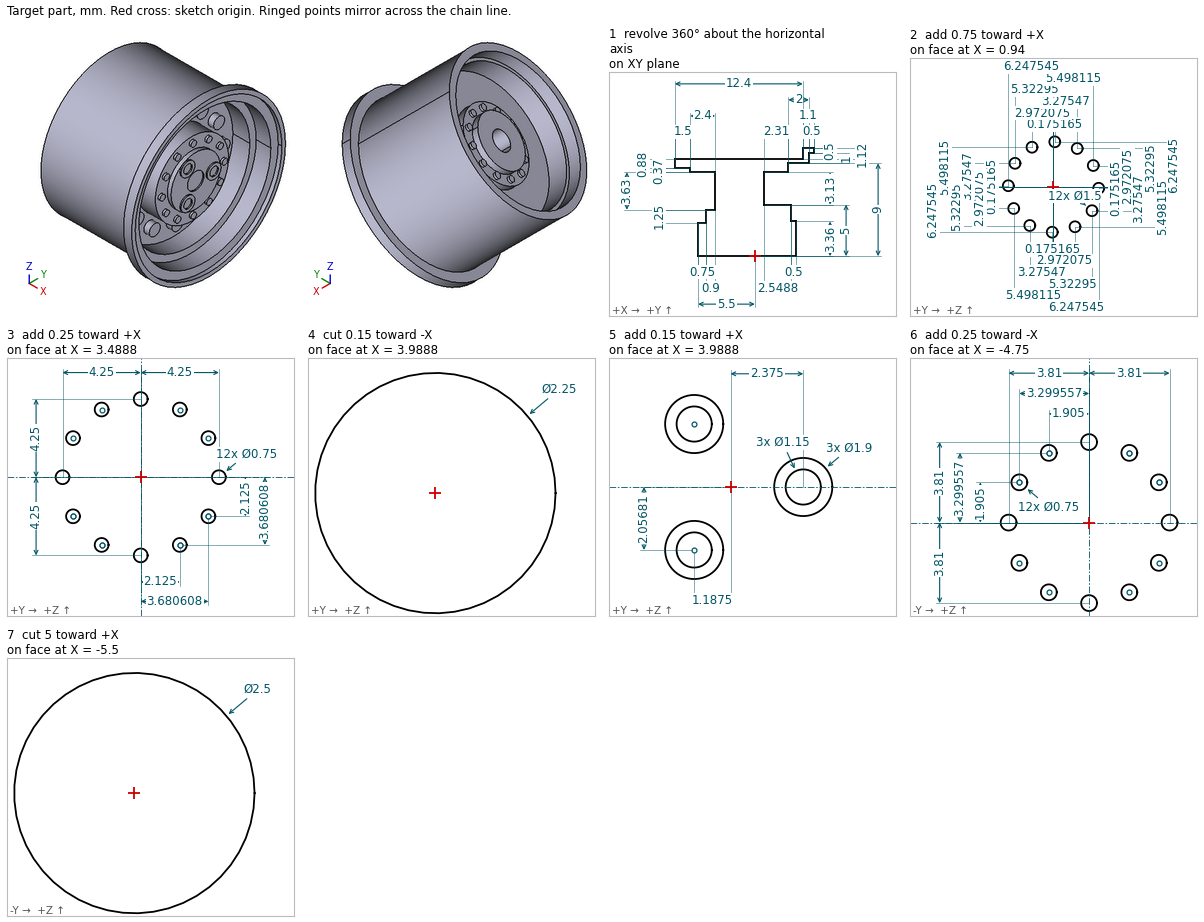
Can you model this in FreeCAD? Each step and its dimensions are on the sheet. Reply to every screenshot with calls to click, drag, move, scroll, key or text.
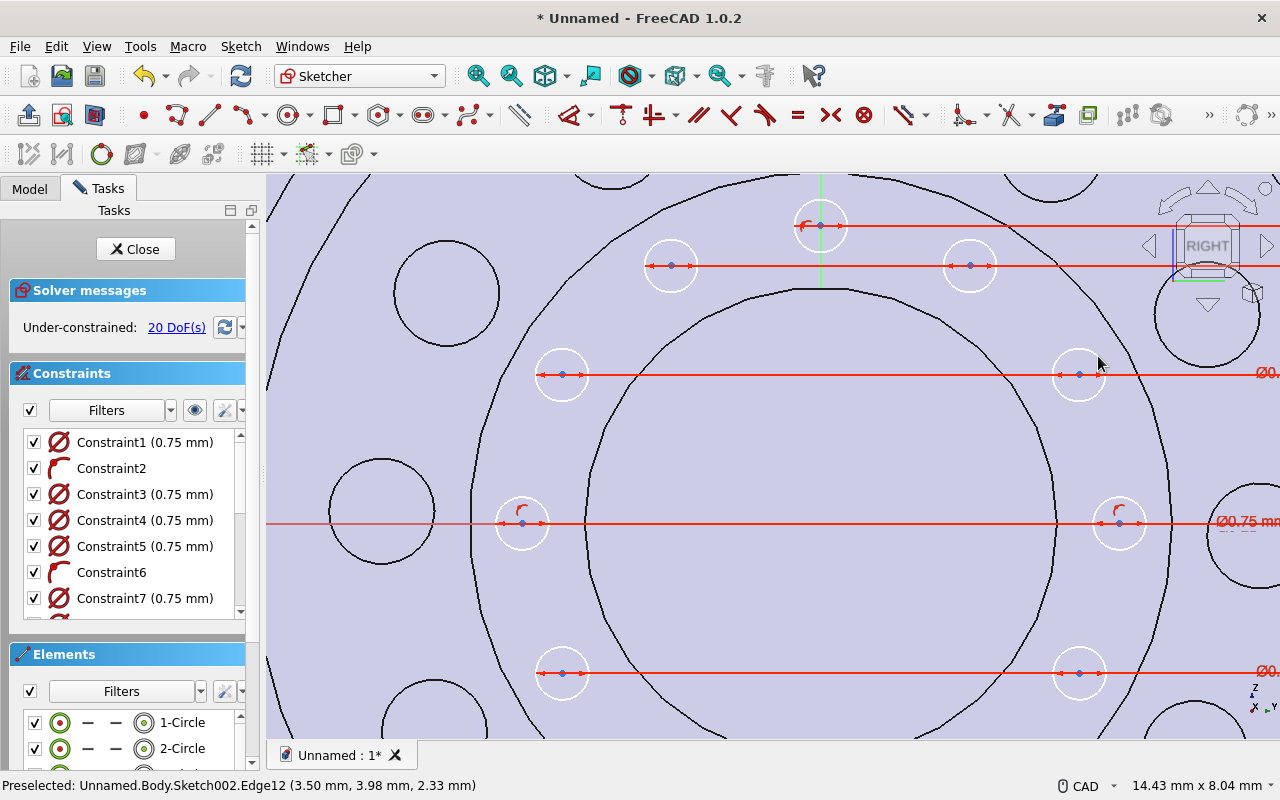
scroll(563, 375, down, 3)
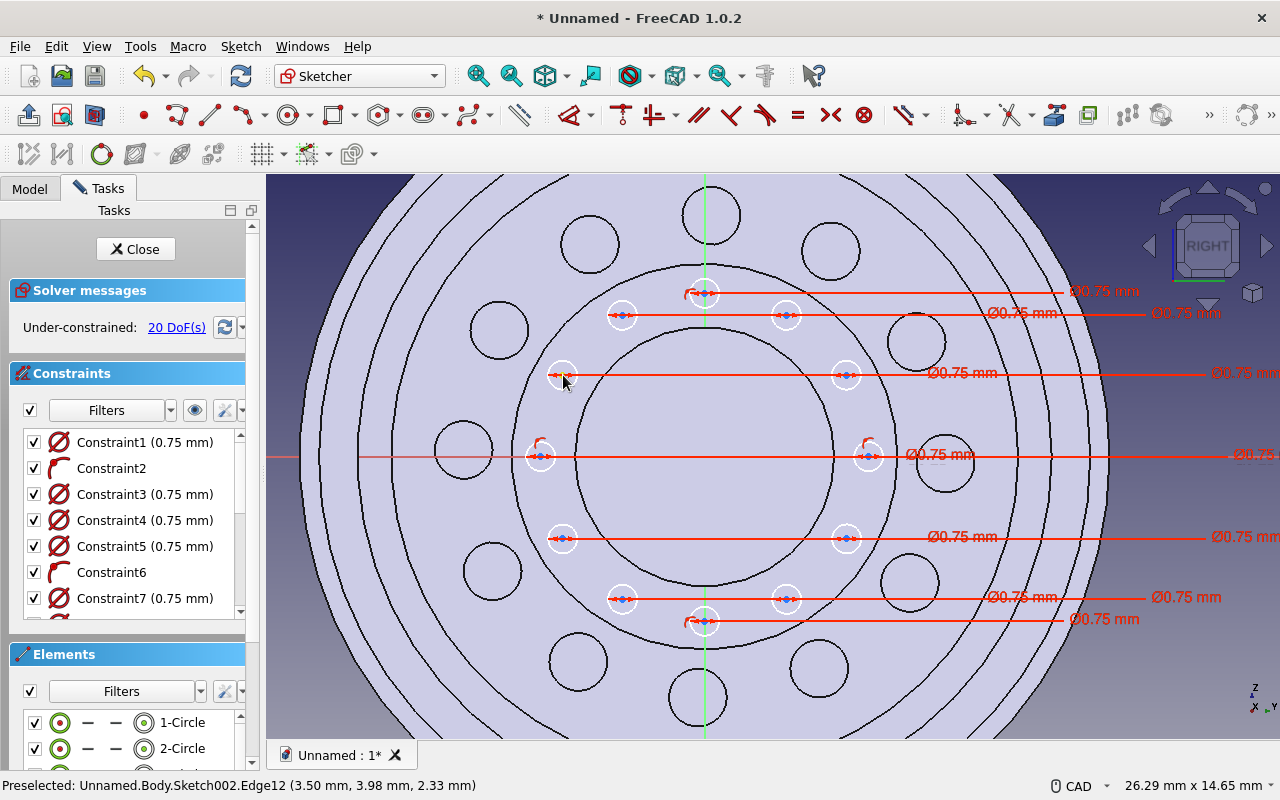
click(787, 599)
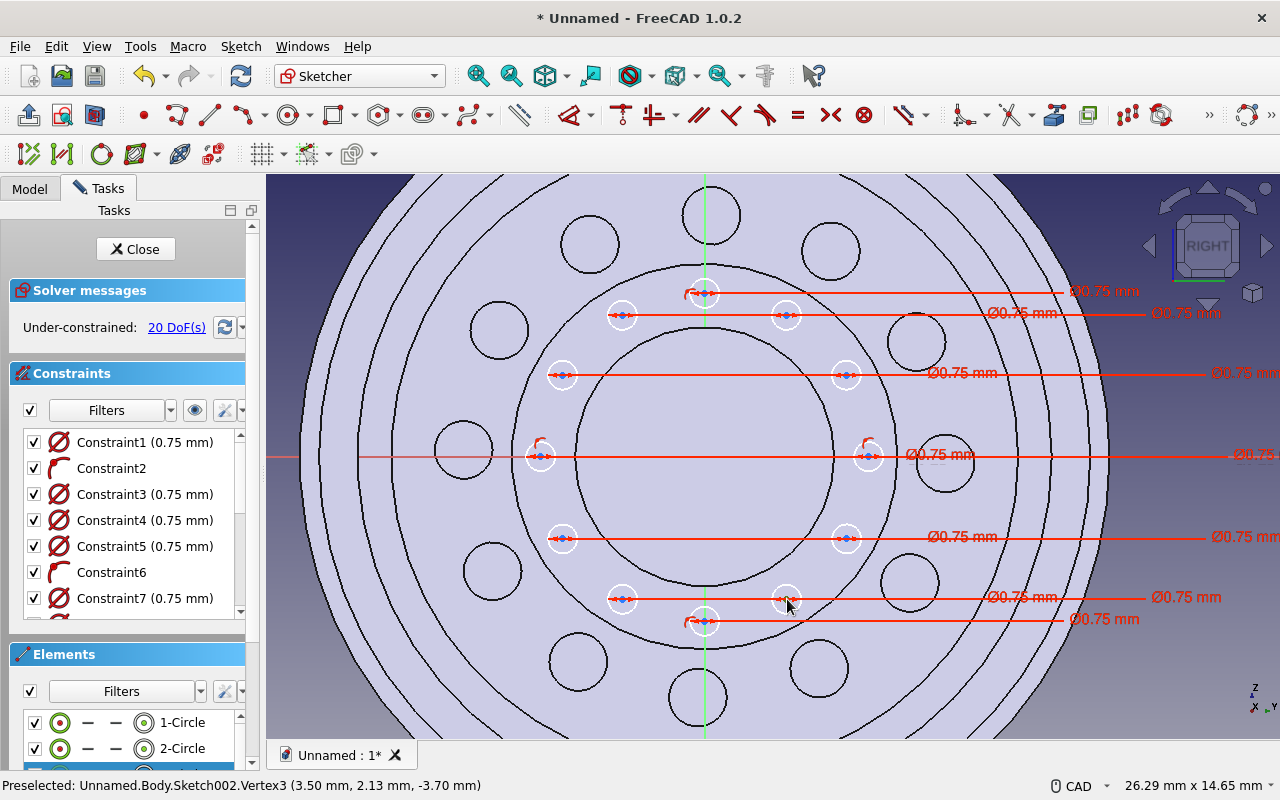
click(623, 599)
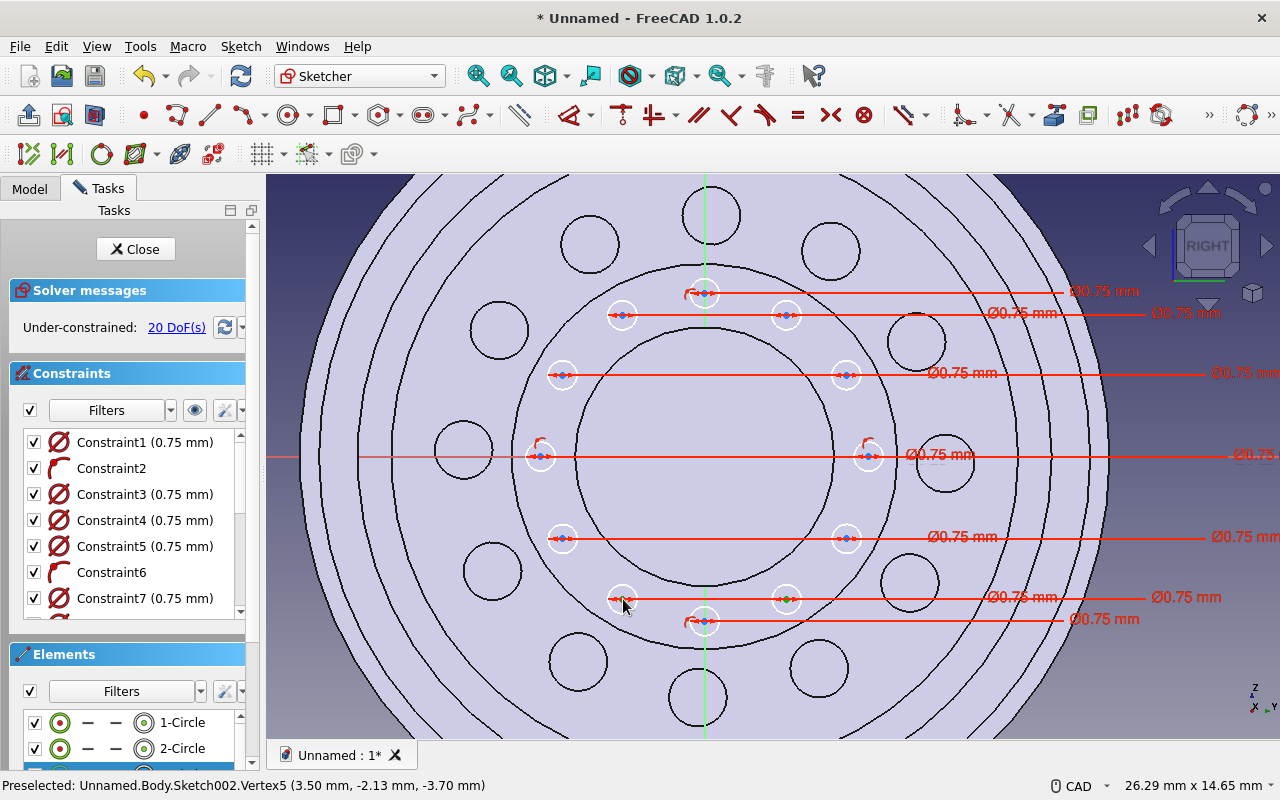
click(705, 675)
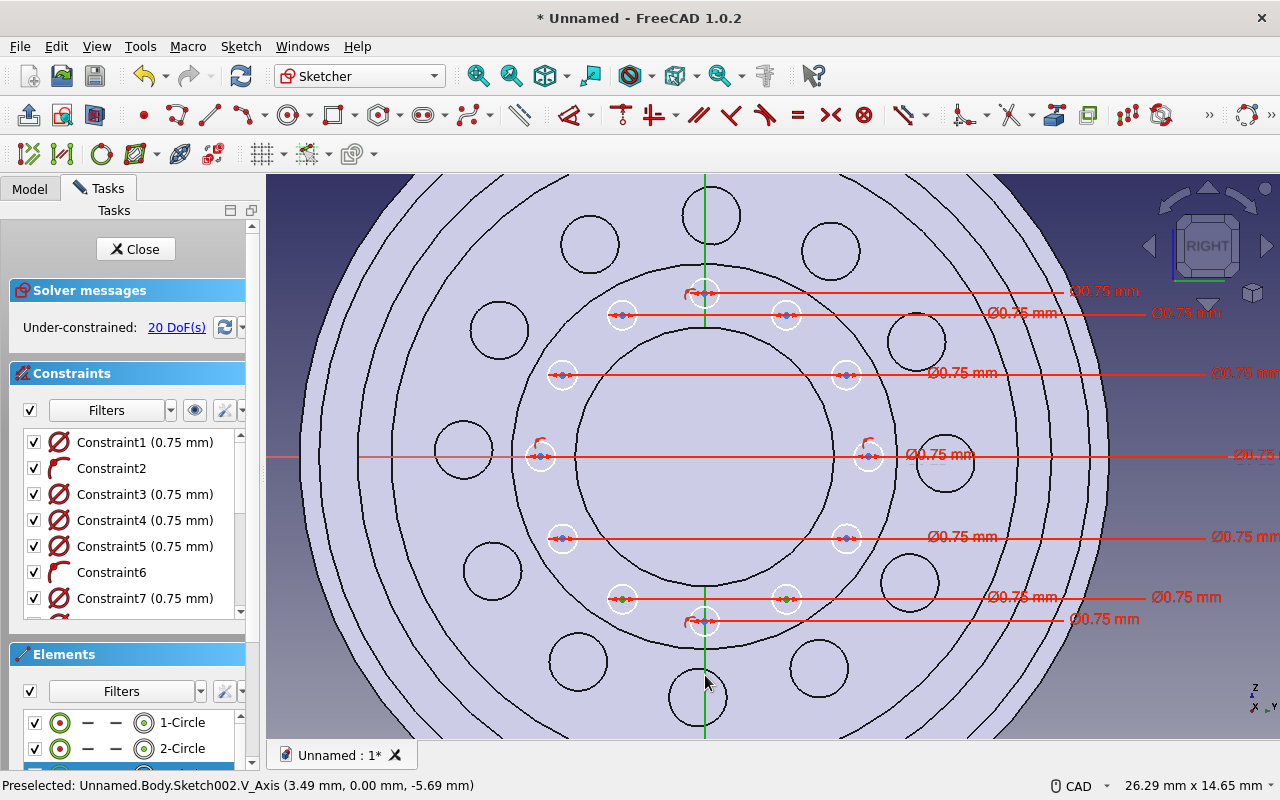
click(831, 116)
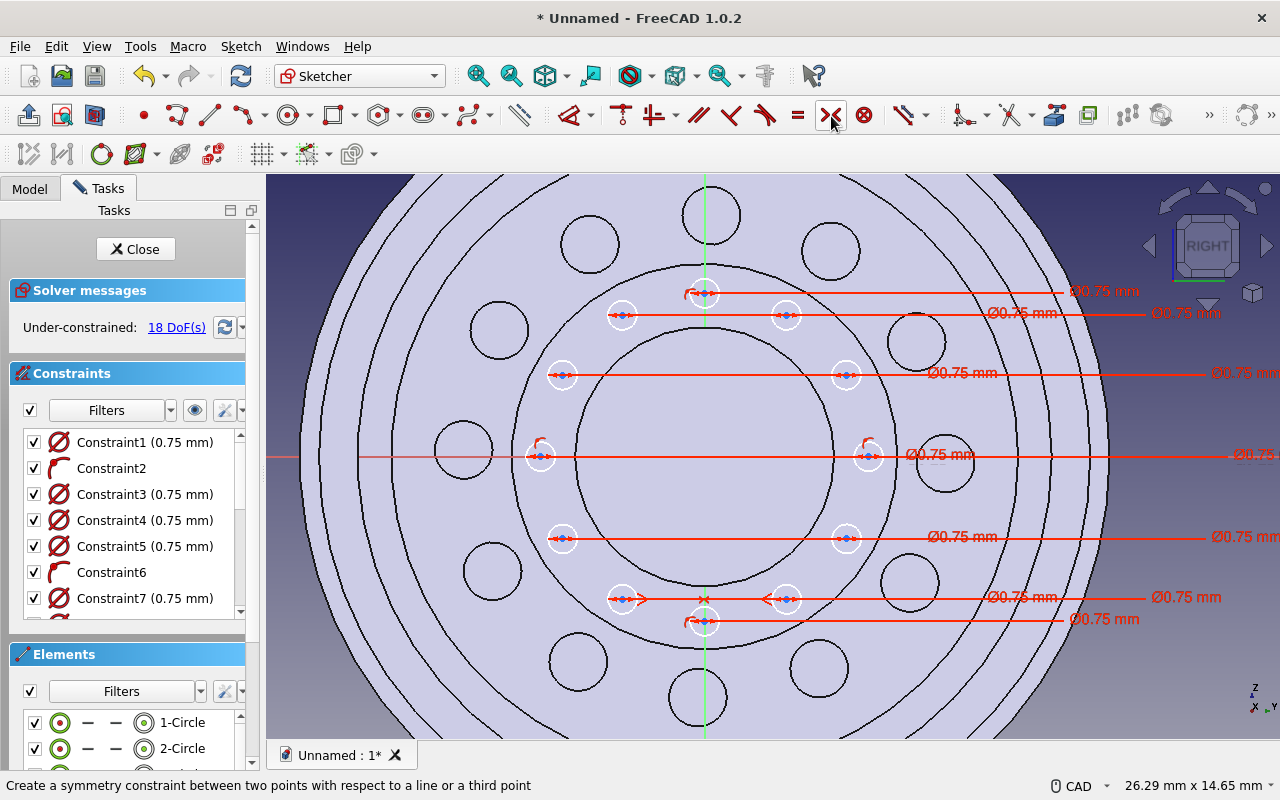
click(847, 539)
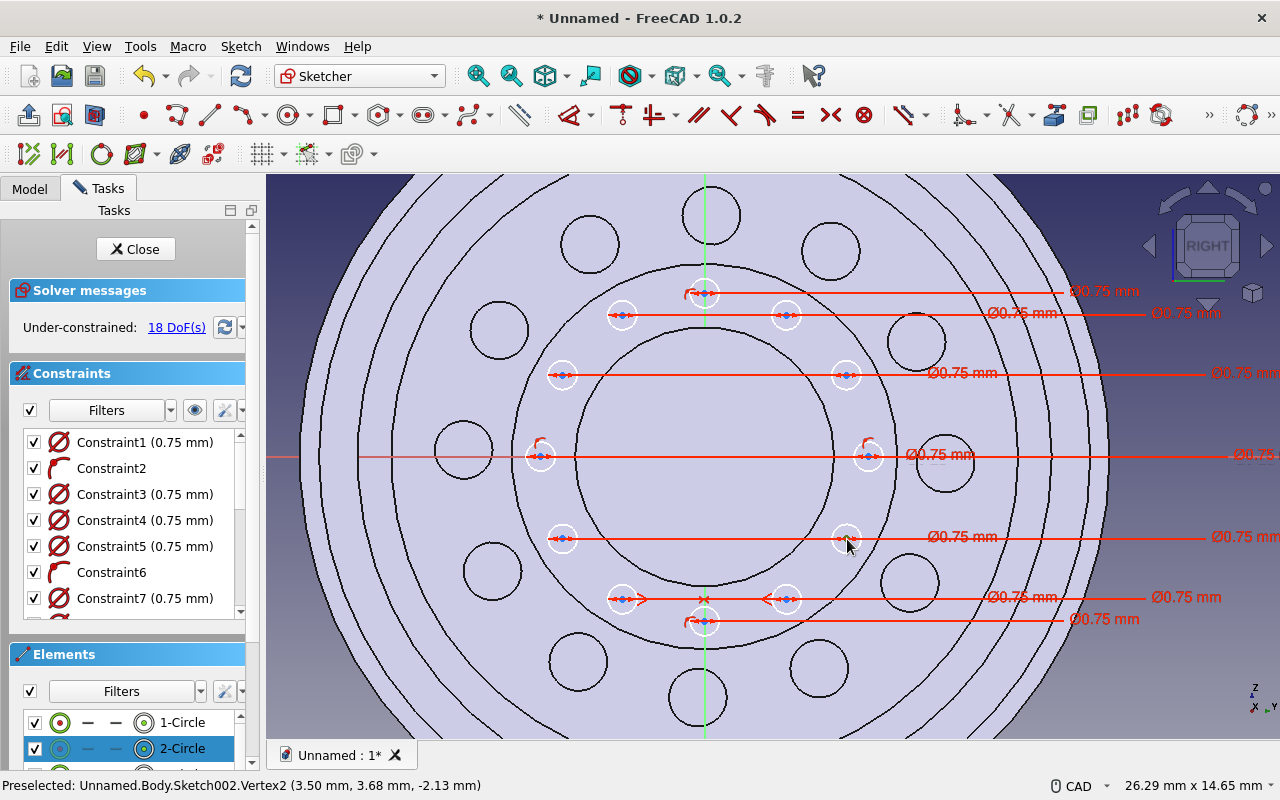
click(563, 539)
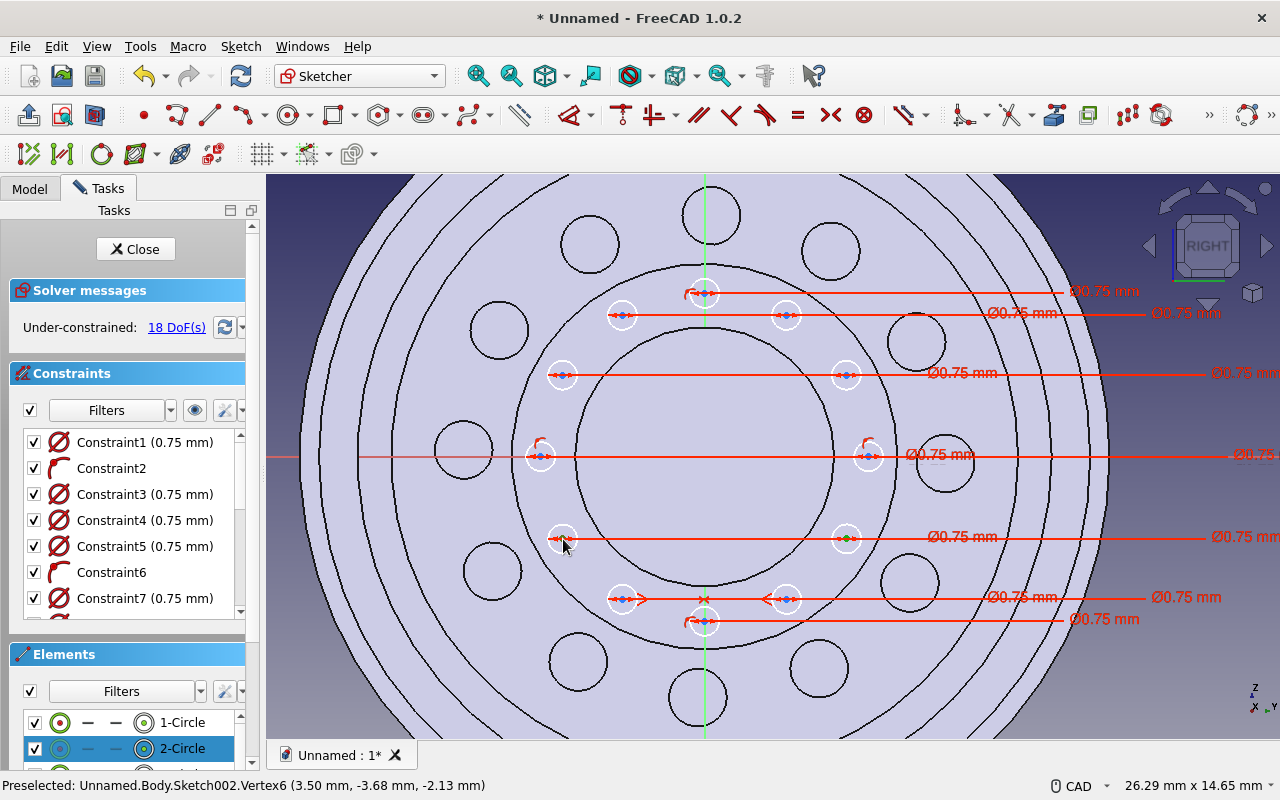
click(705, 675)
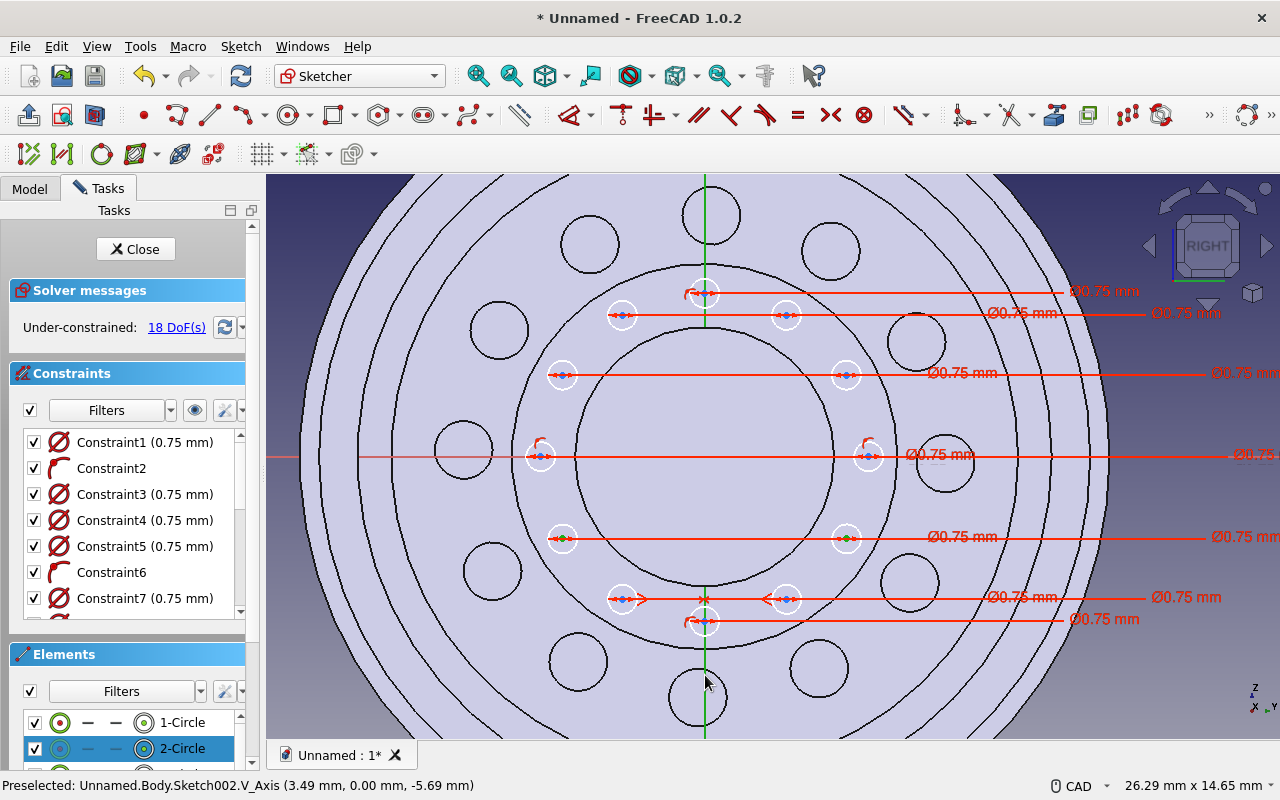
click(831, 116)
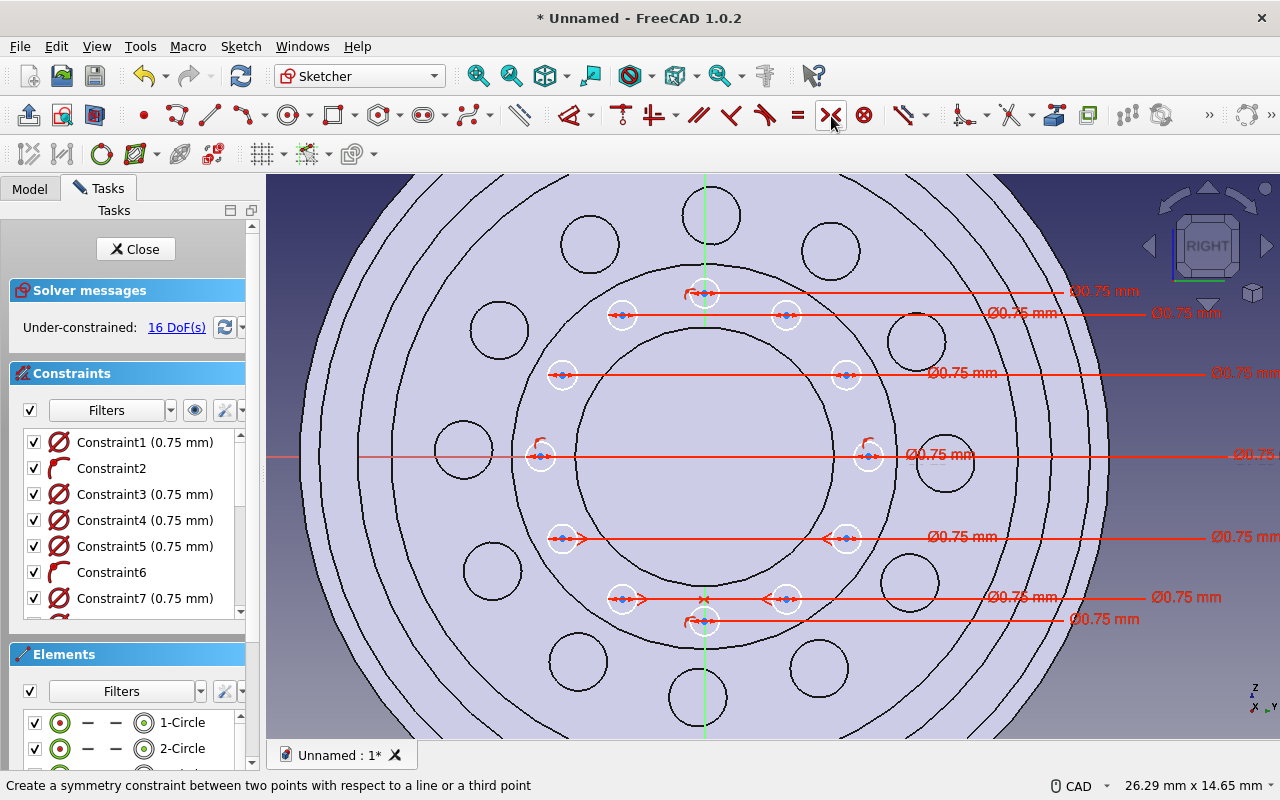
click(563, 539)